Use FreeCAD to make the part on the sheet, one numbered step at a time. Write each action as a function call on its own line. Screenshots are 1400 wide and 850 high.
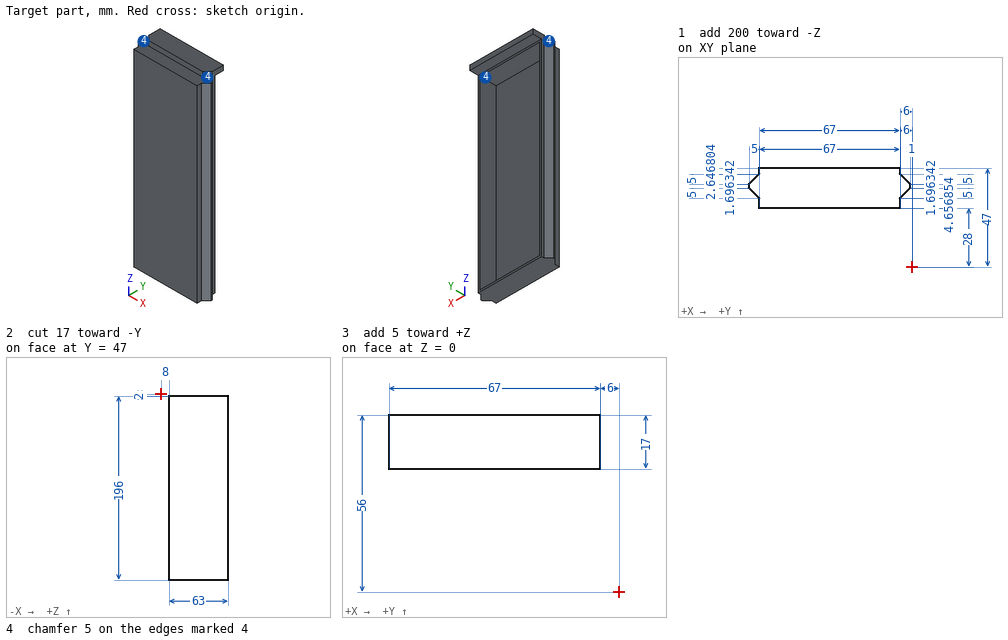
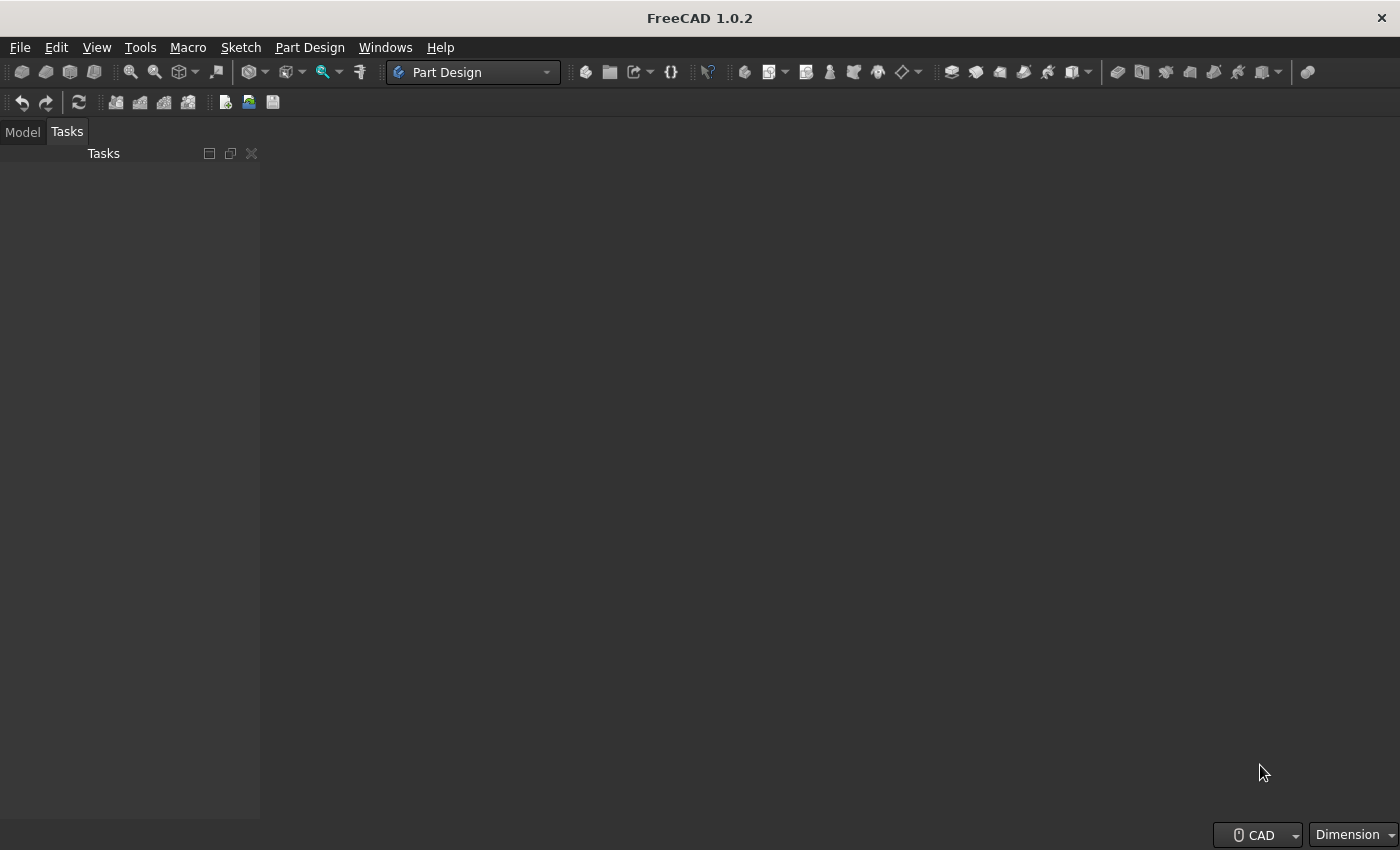
click(226, 102)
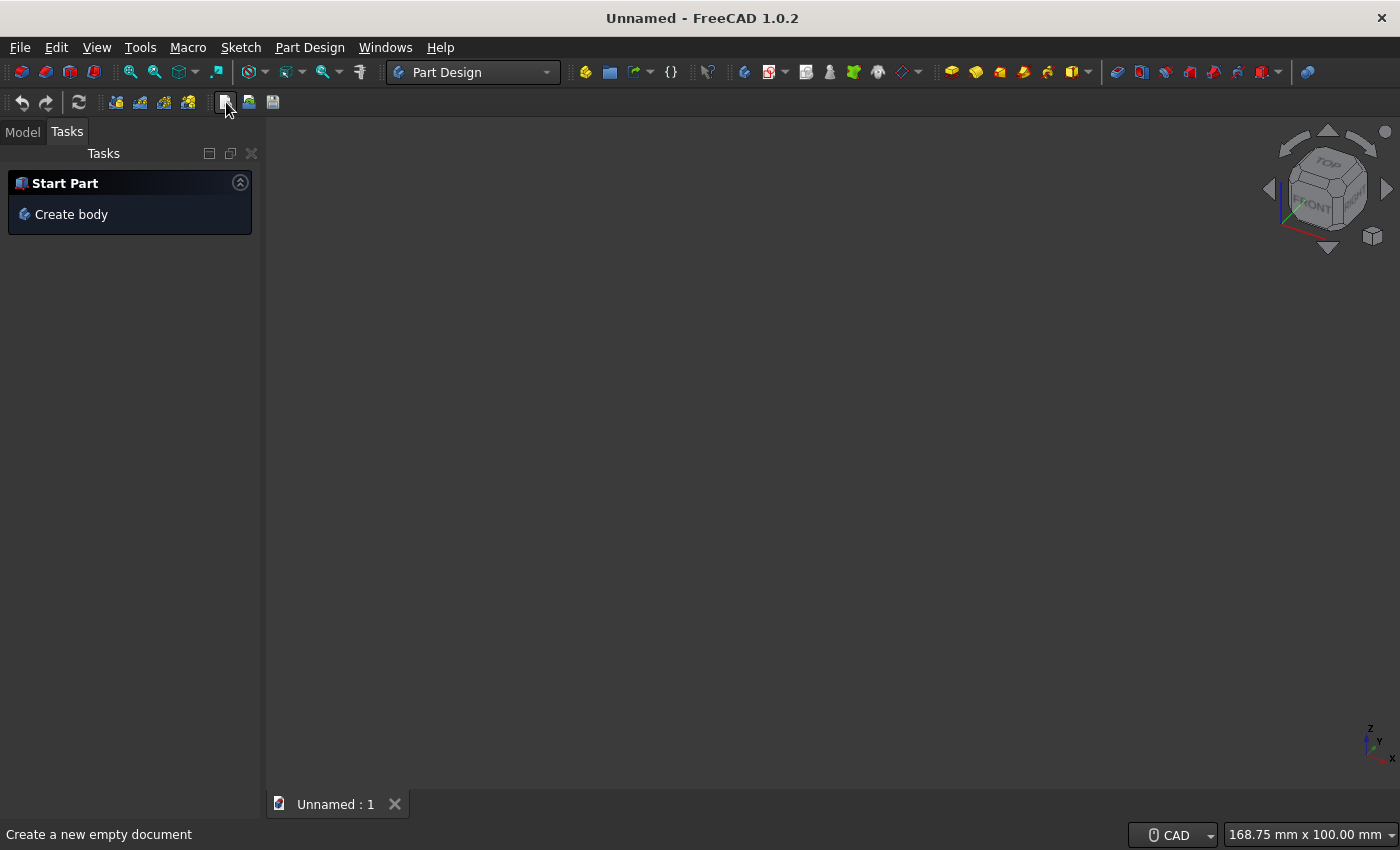
click(770, 72)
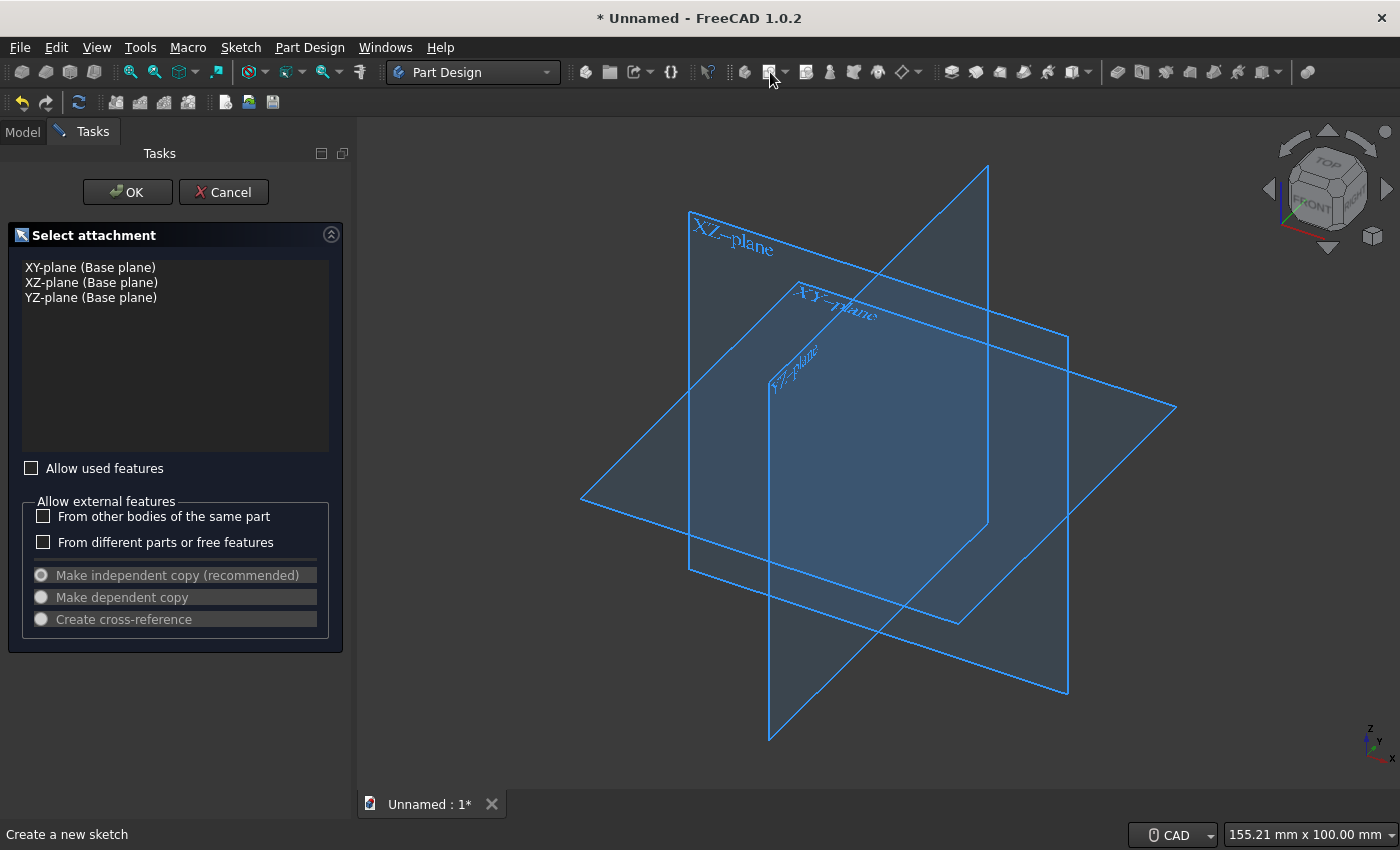
click(82, 268)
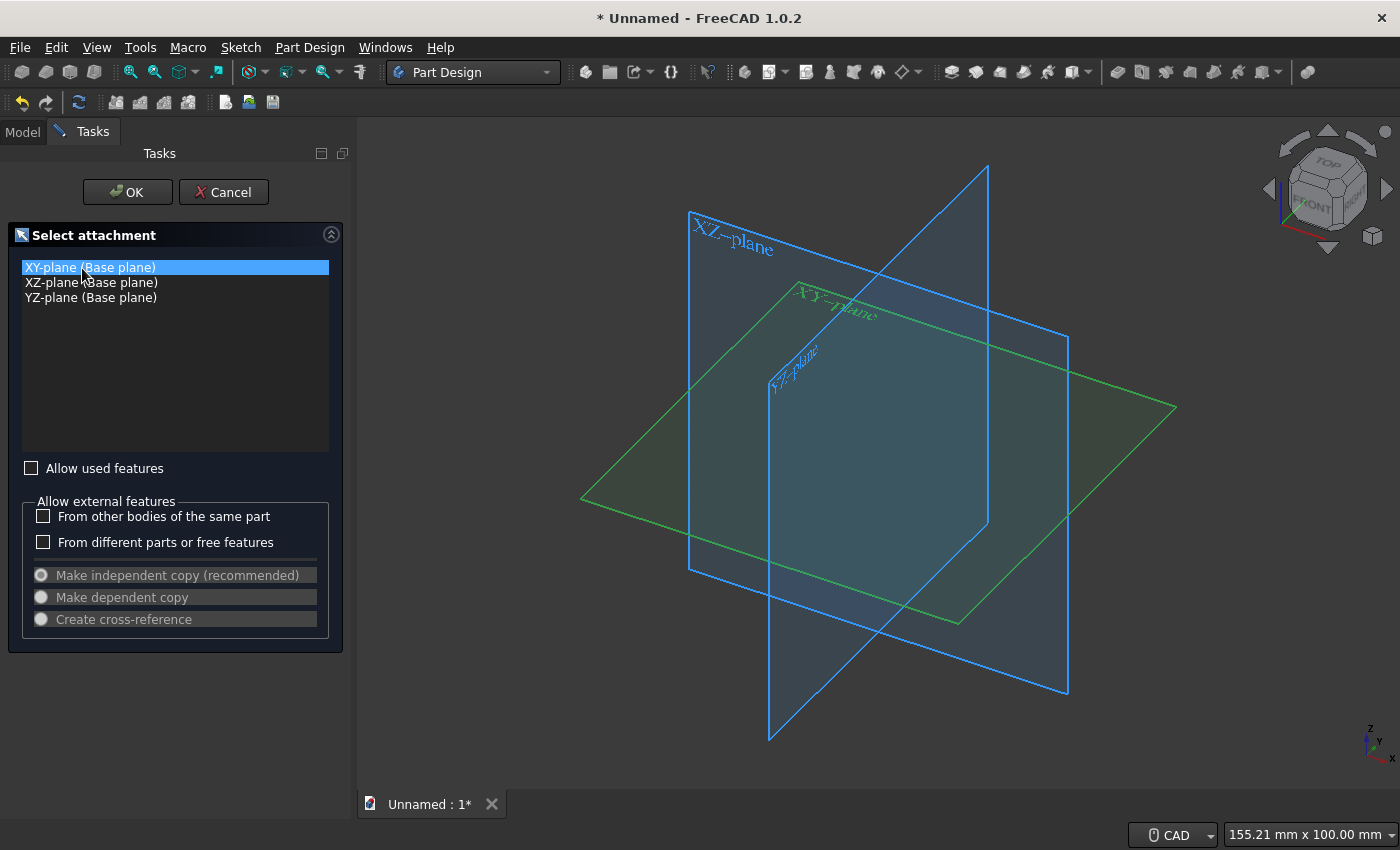
click(128, 192)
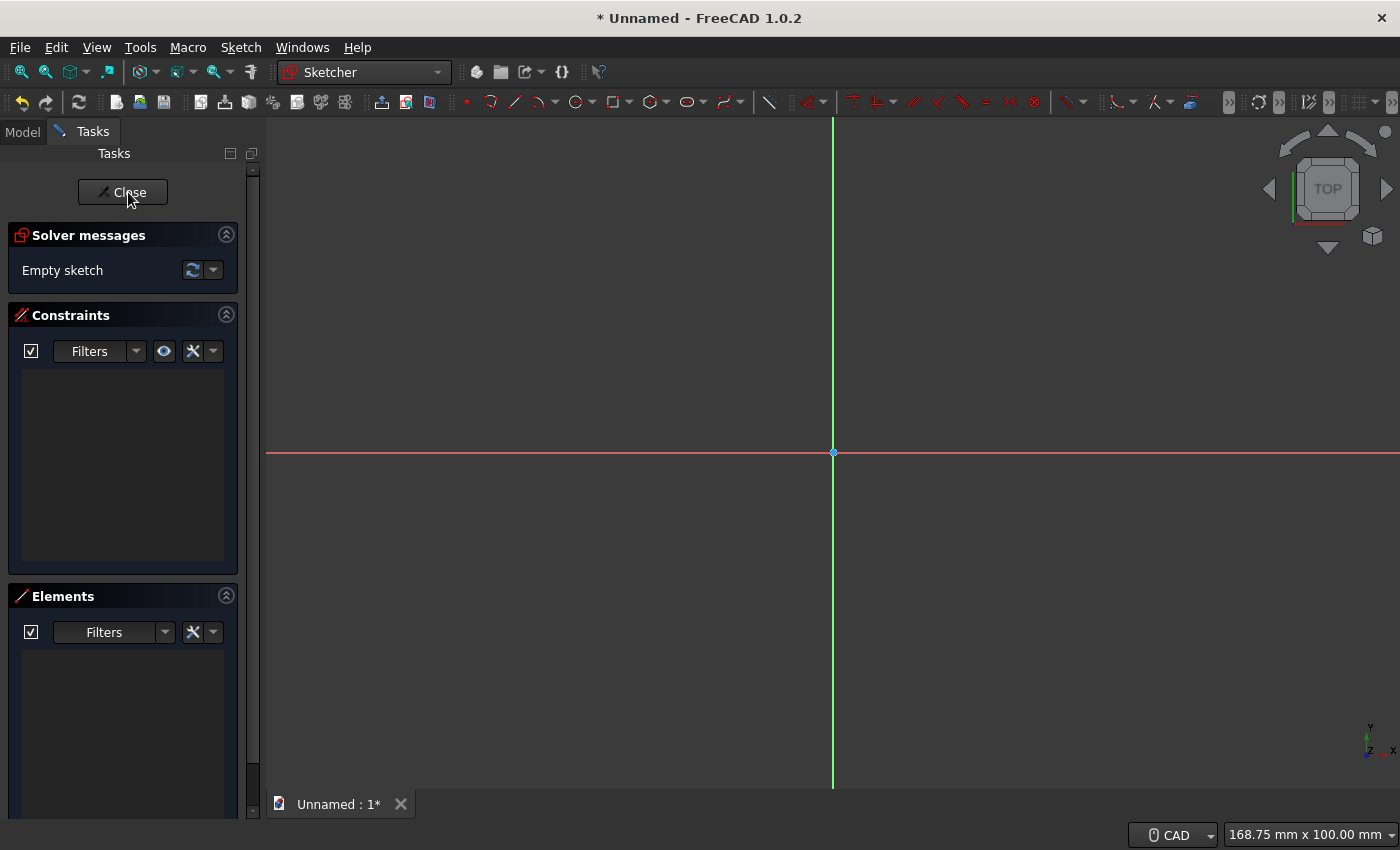
scroll(1235, 761, down, 1)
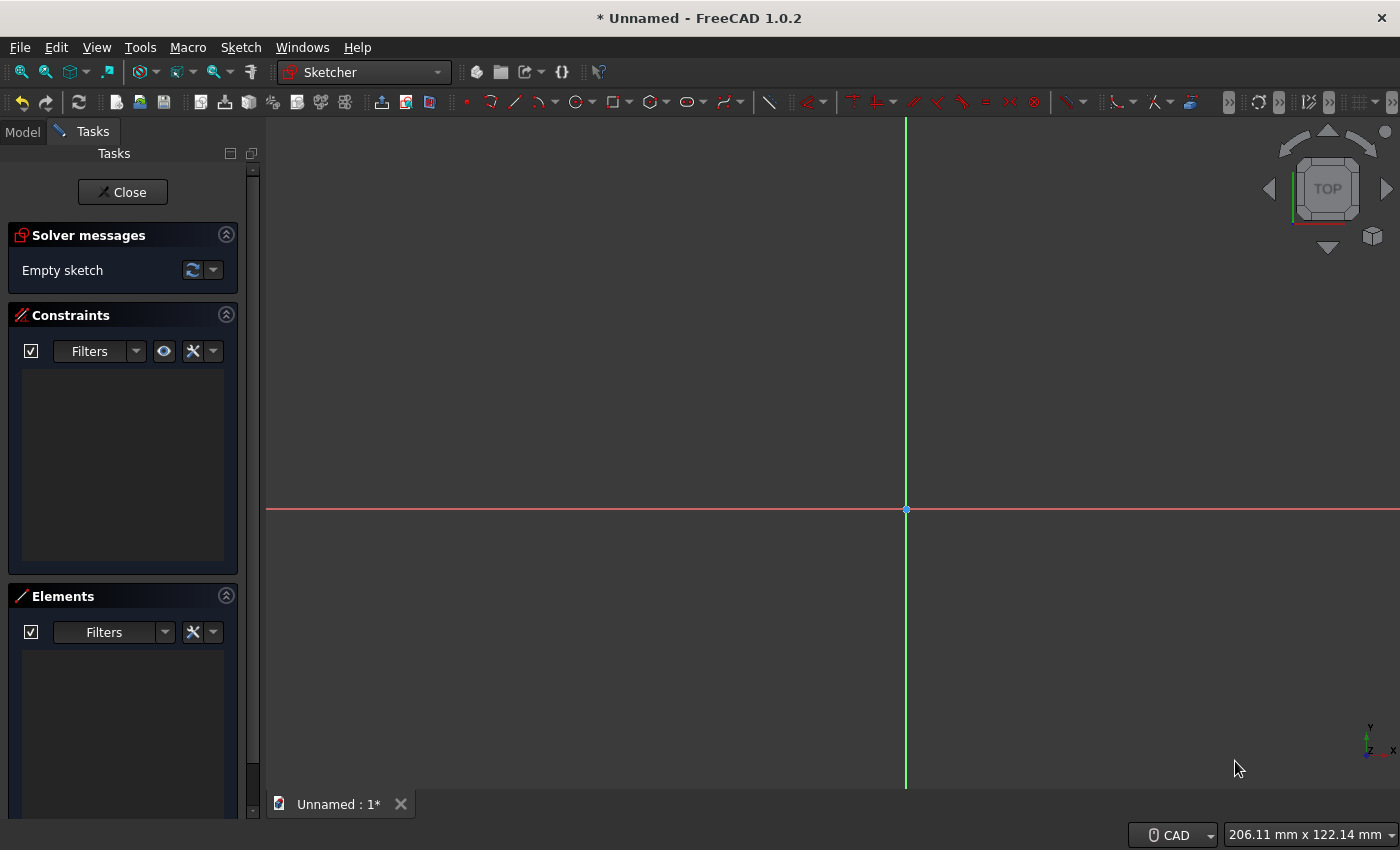
scroll(543, 231, up, 2)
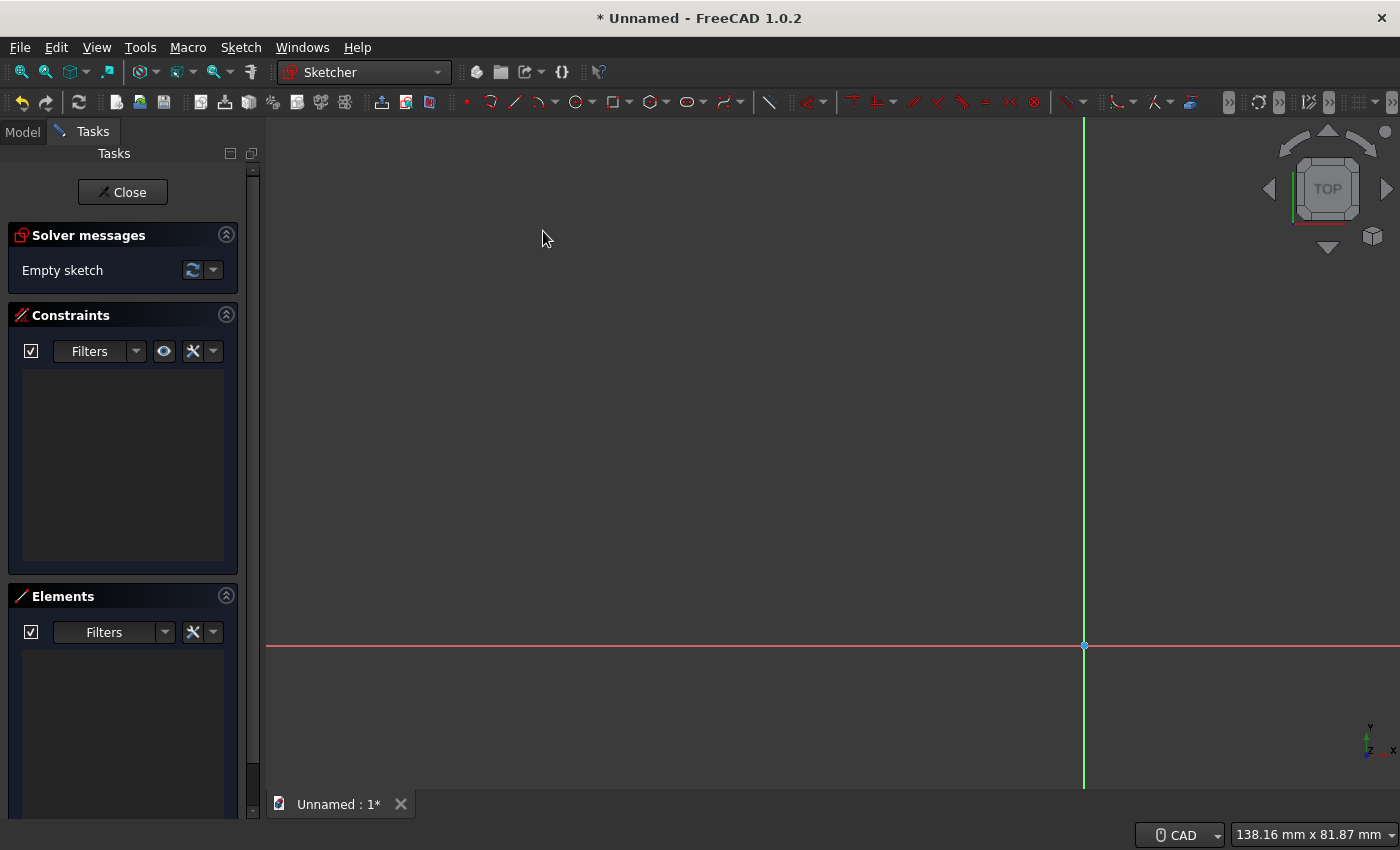
click(492, 102)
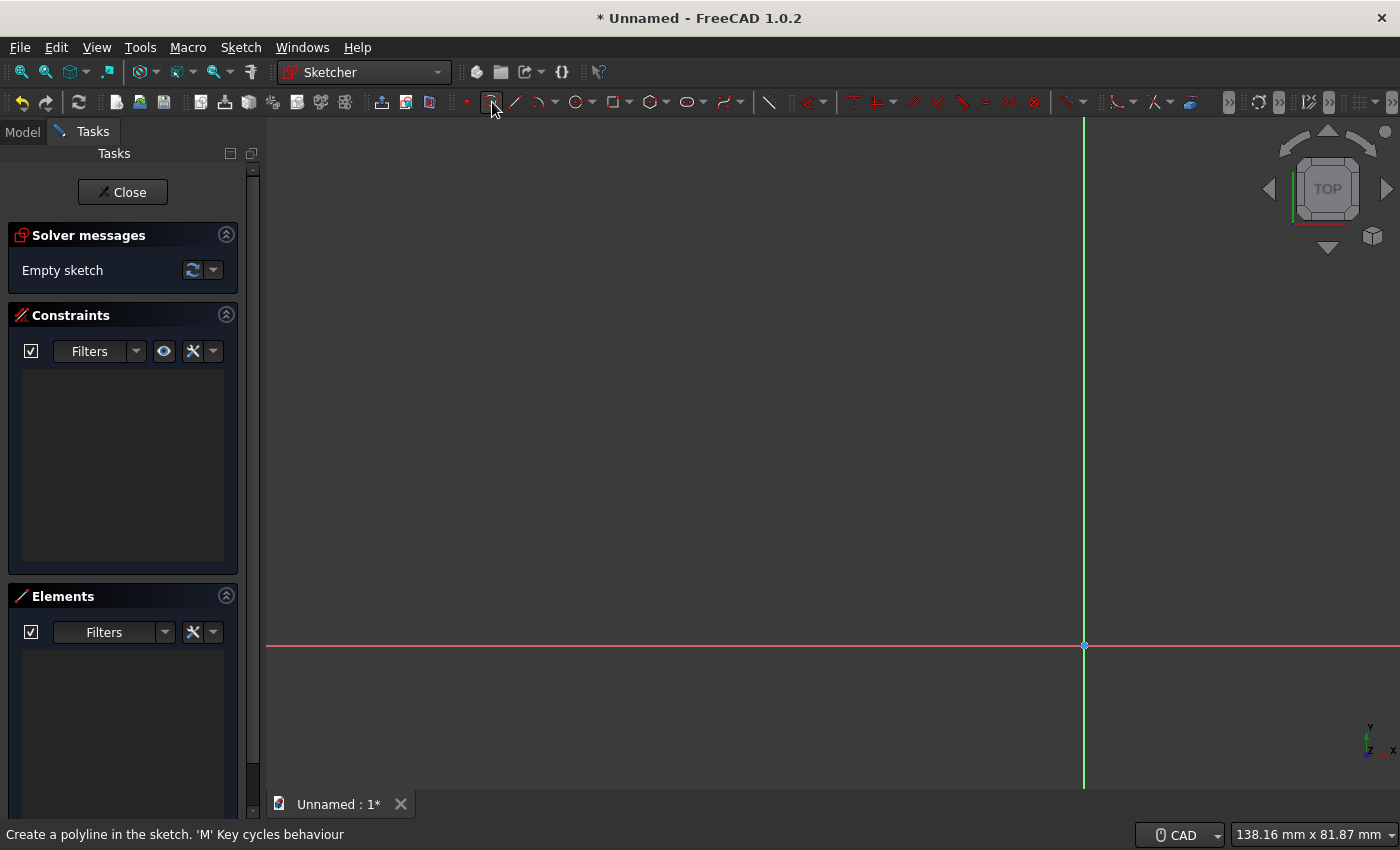
click(1035, 416)
click(1035, 378)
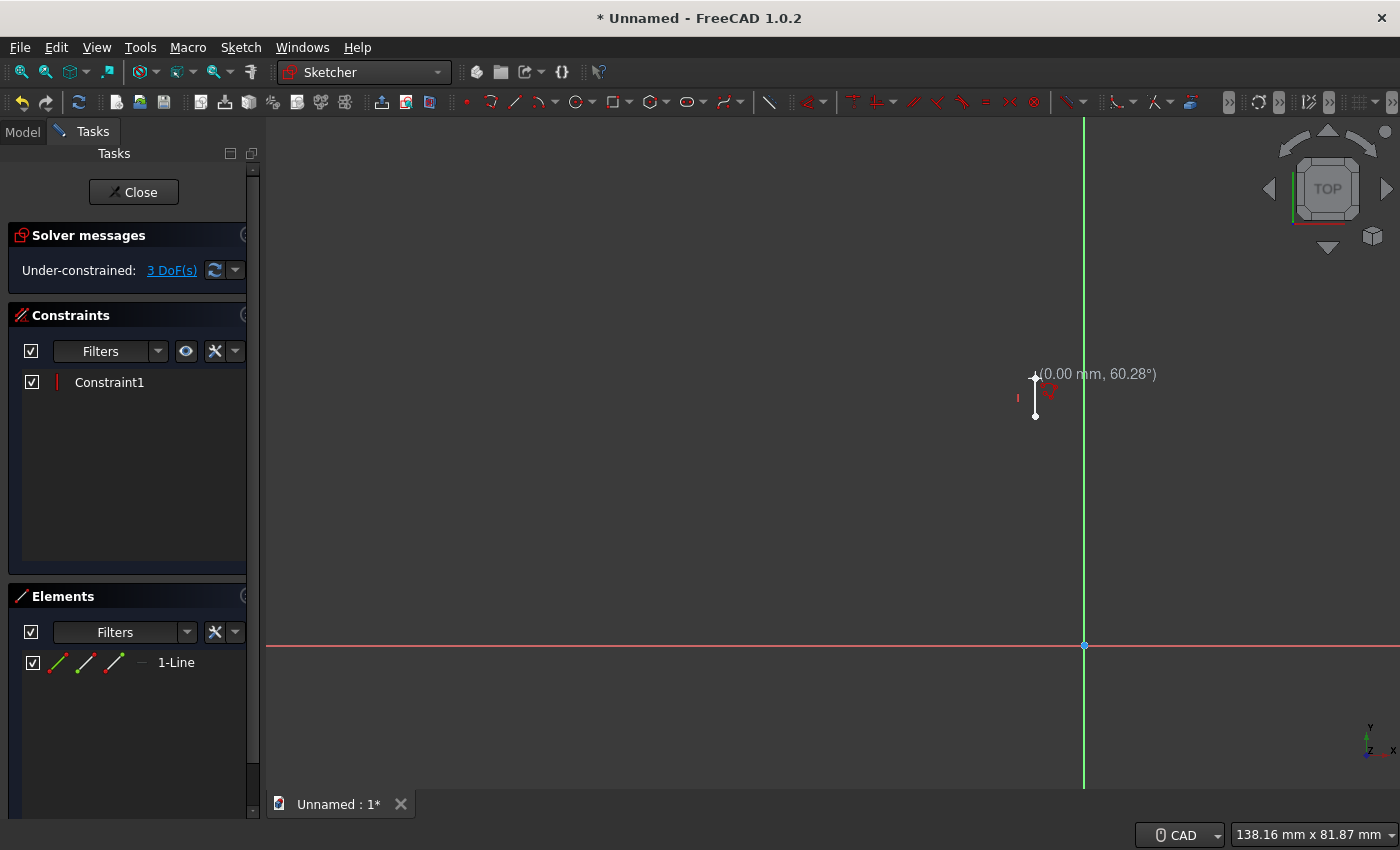
scroll(1076, 337, up, 4)